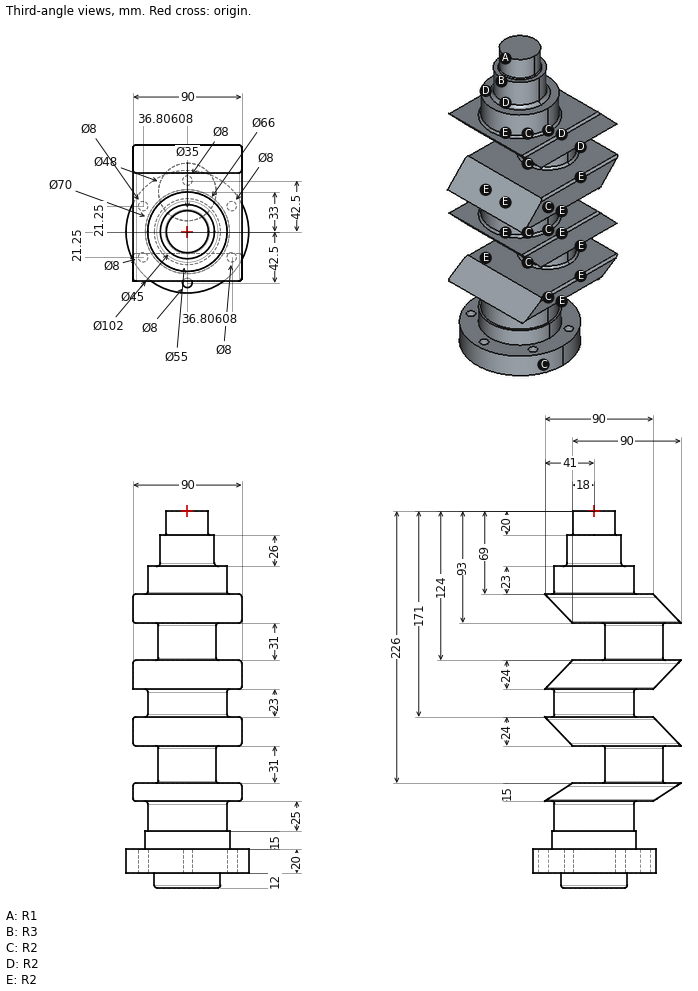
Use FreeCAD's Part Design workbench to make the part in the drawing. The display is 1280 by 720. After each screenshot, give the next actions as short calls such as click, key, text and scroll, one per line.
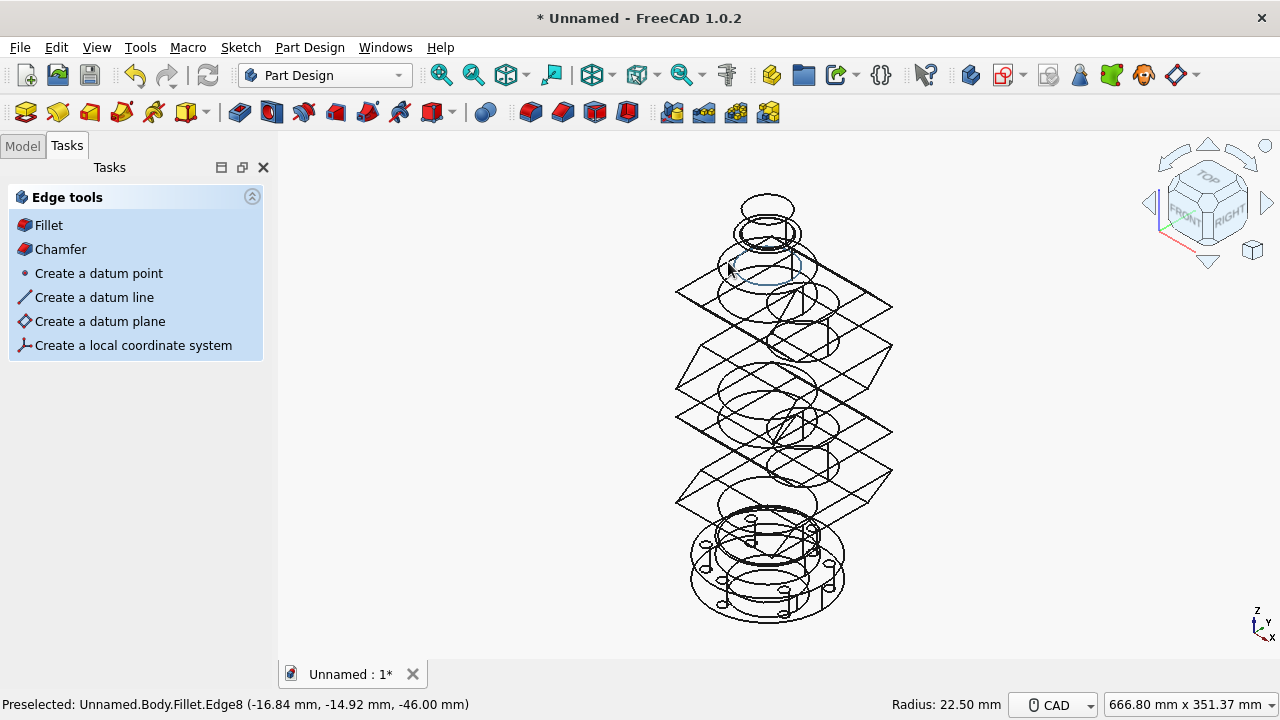
key(v)
key(1)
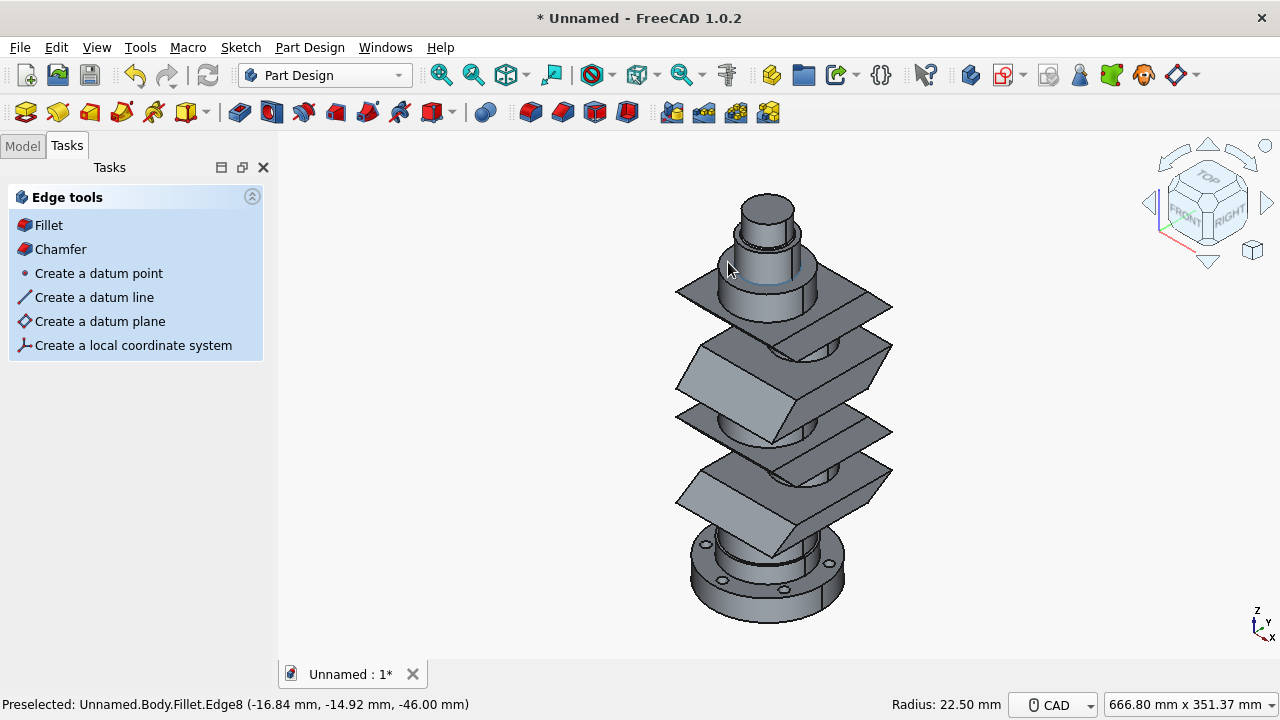
click(532, 112)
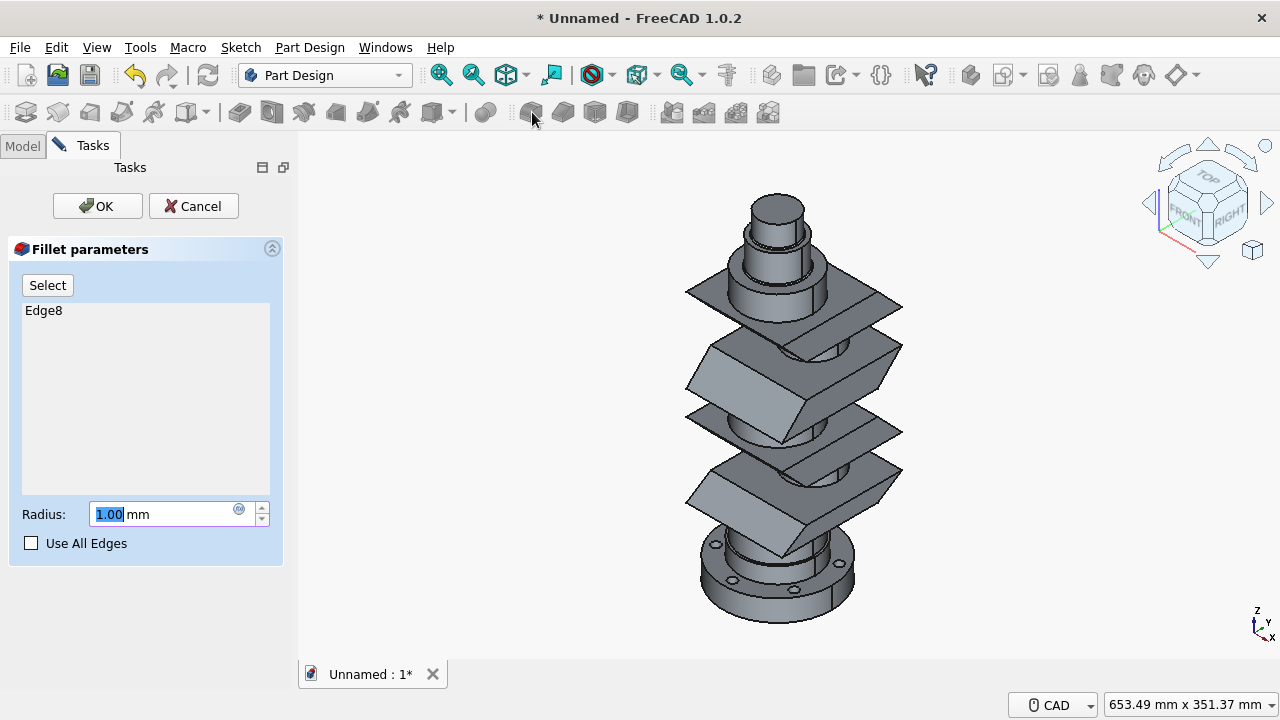
text(3)
key(Tab)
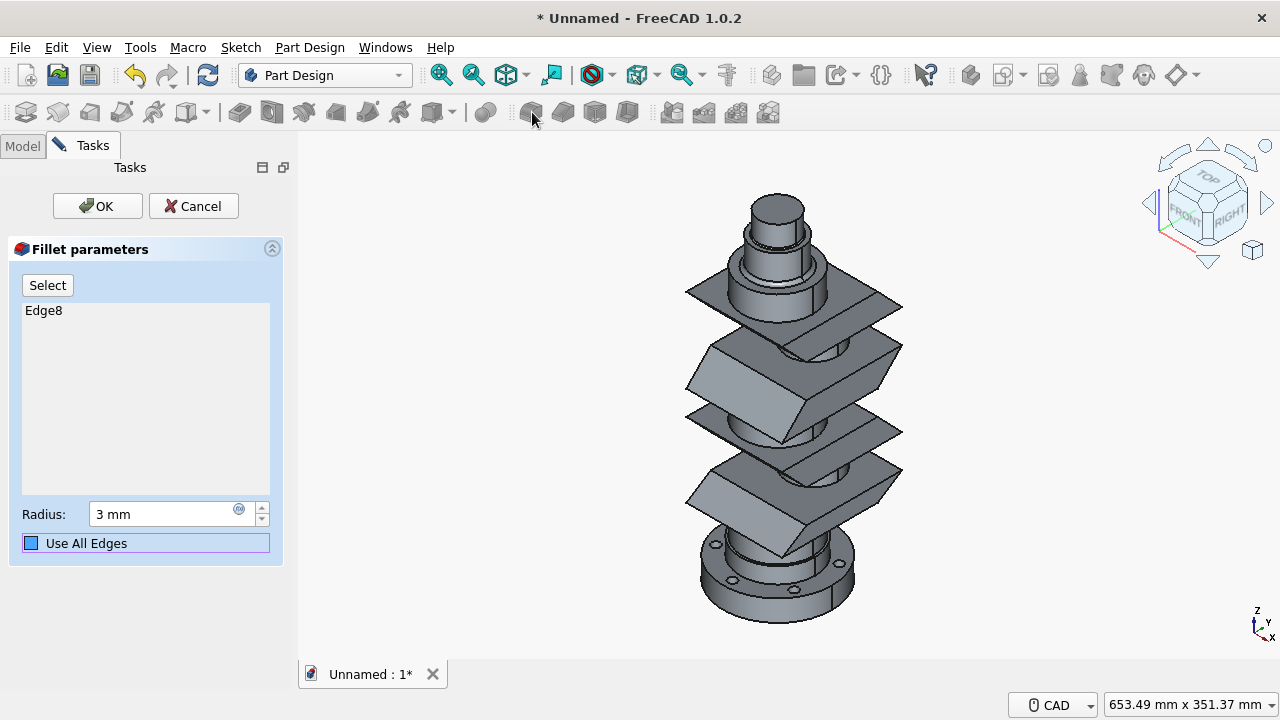
click(98, 206)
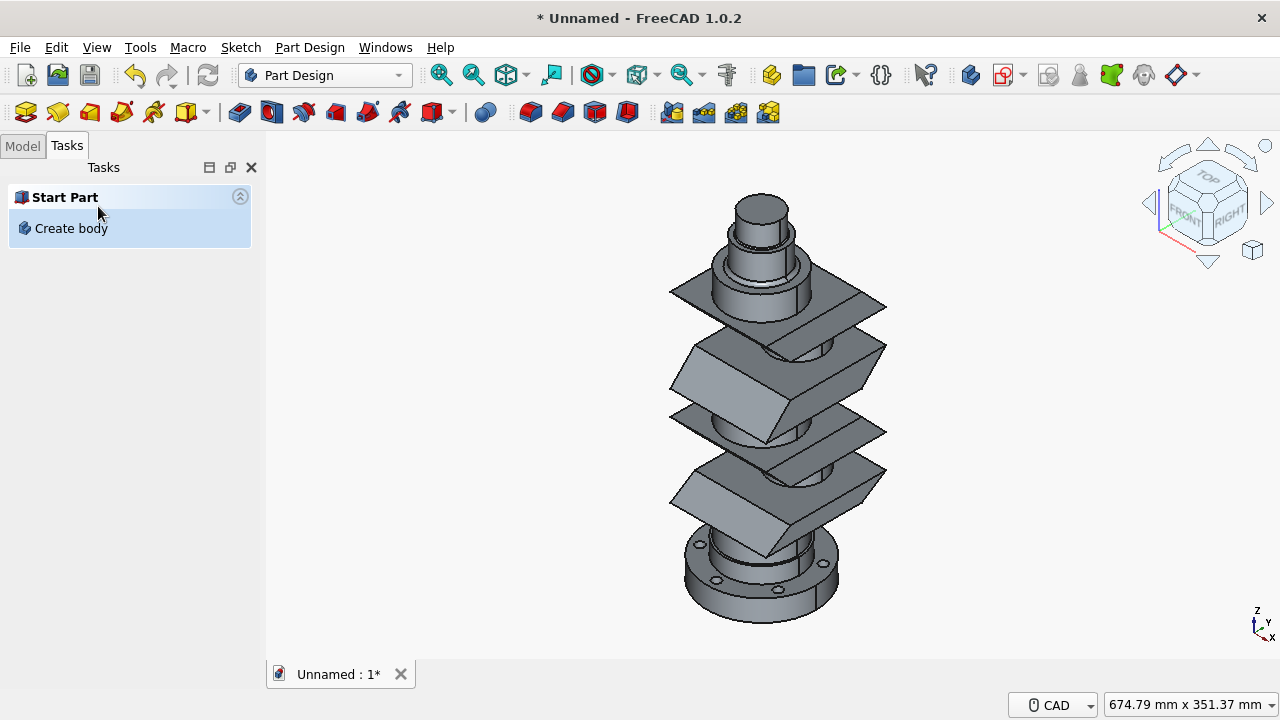
key(2)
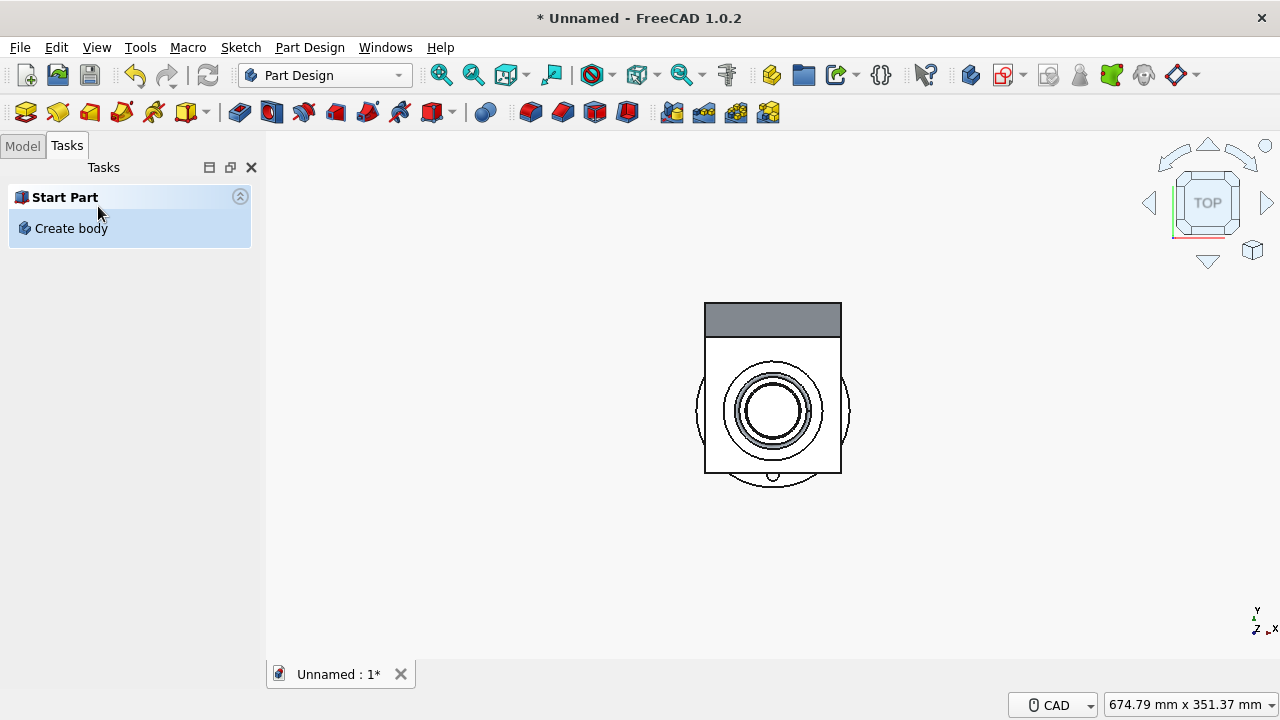
click(442, 76)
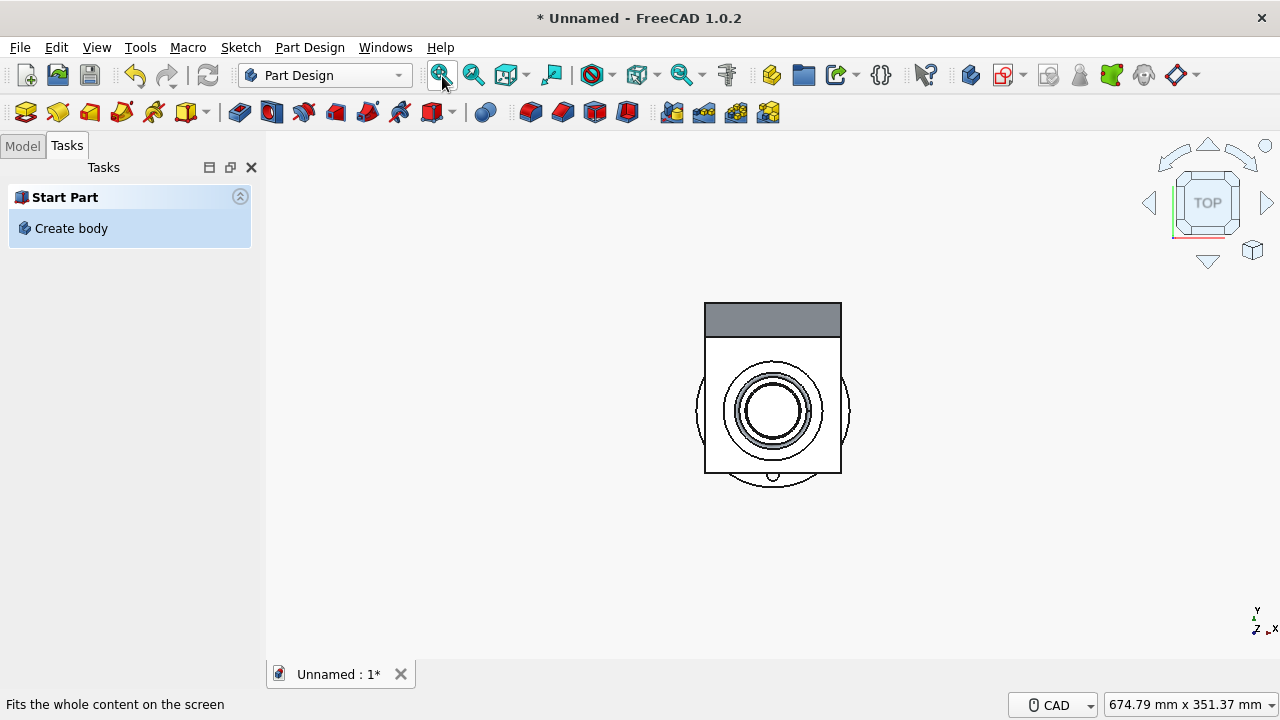
key(0)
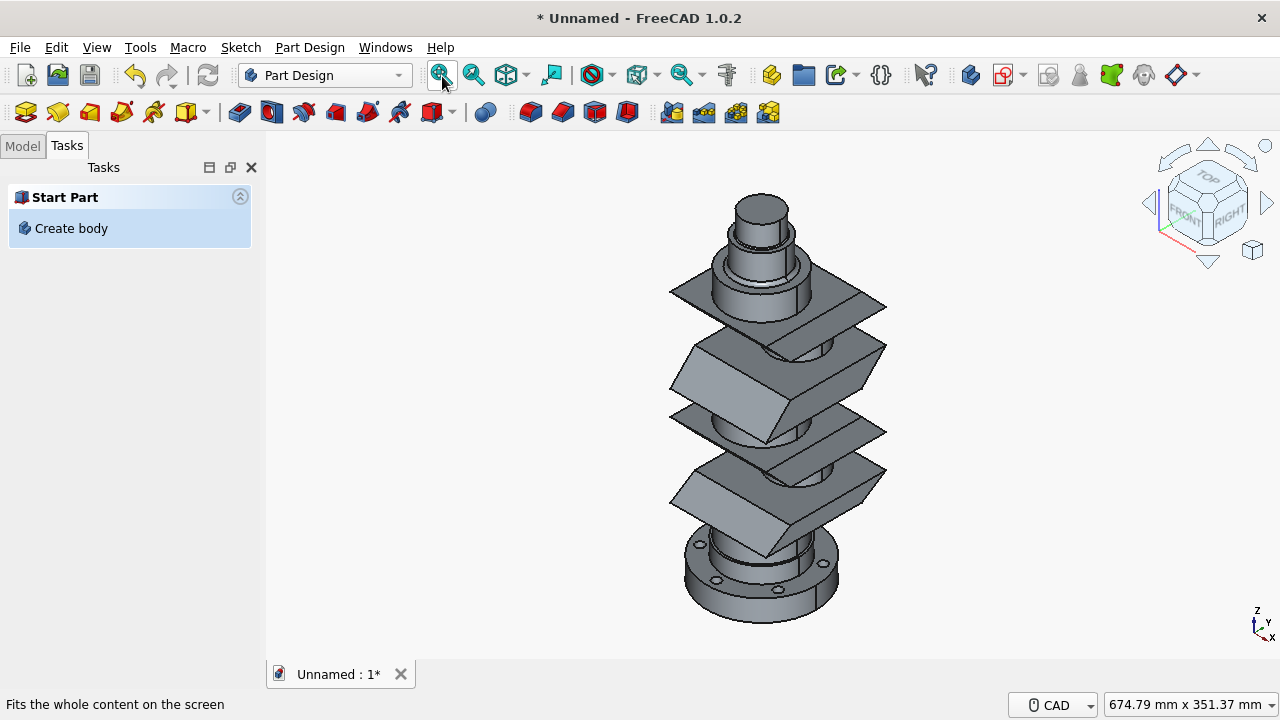
key(1)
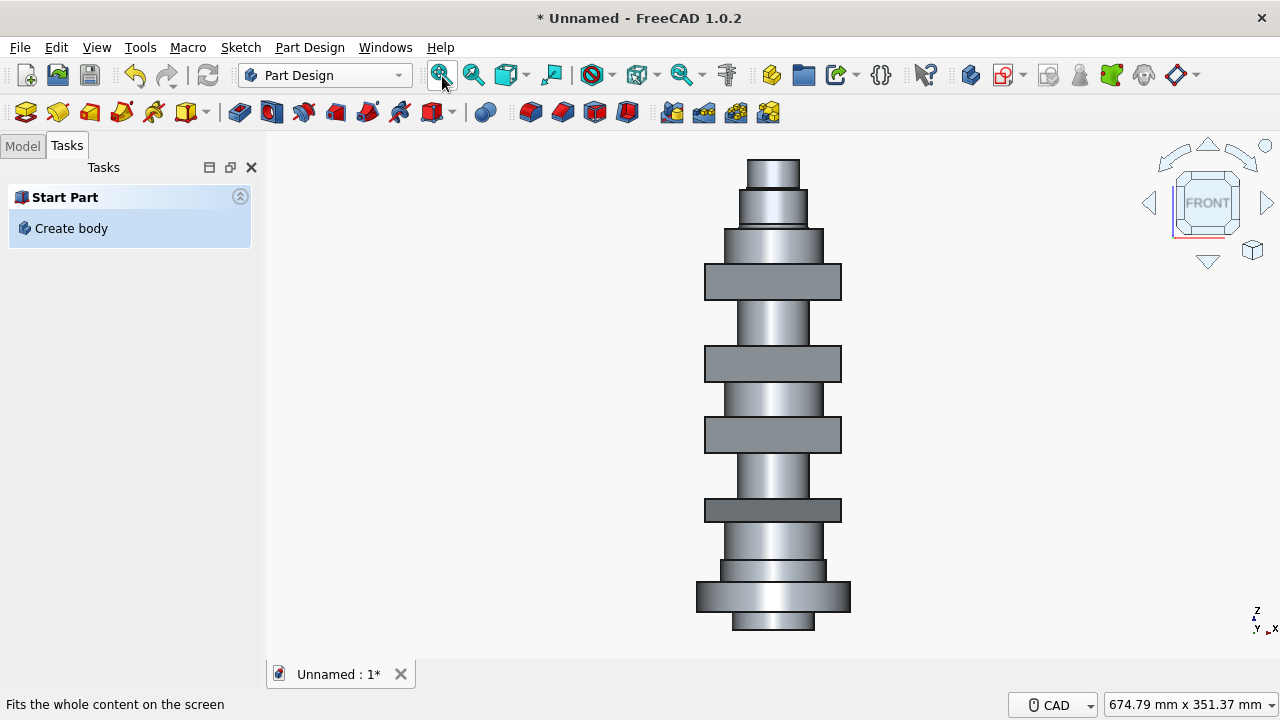
click(740, 629)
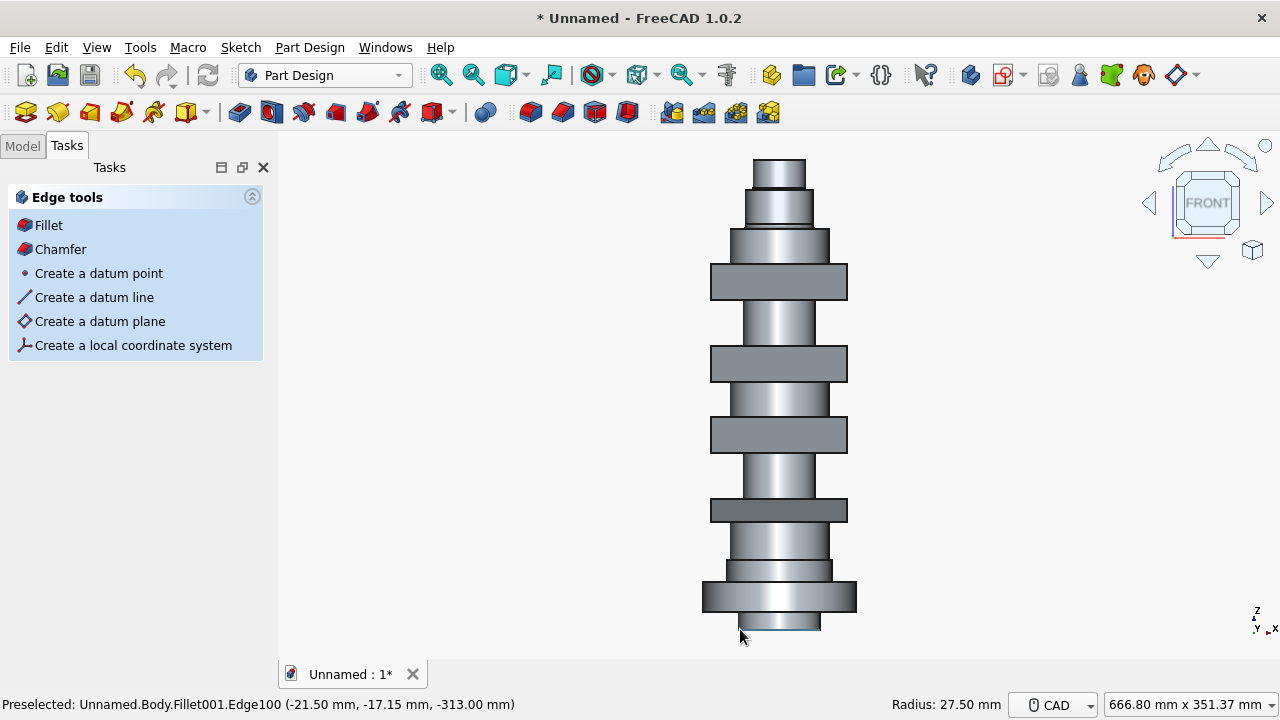
key(3)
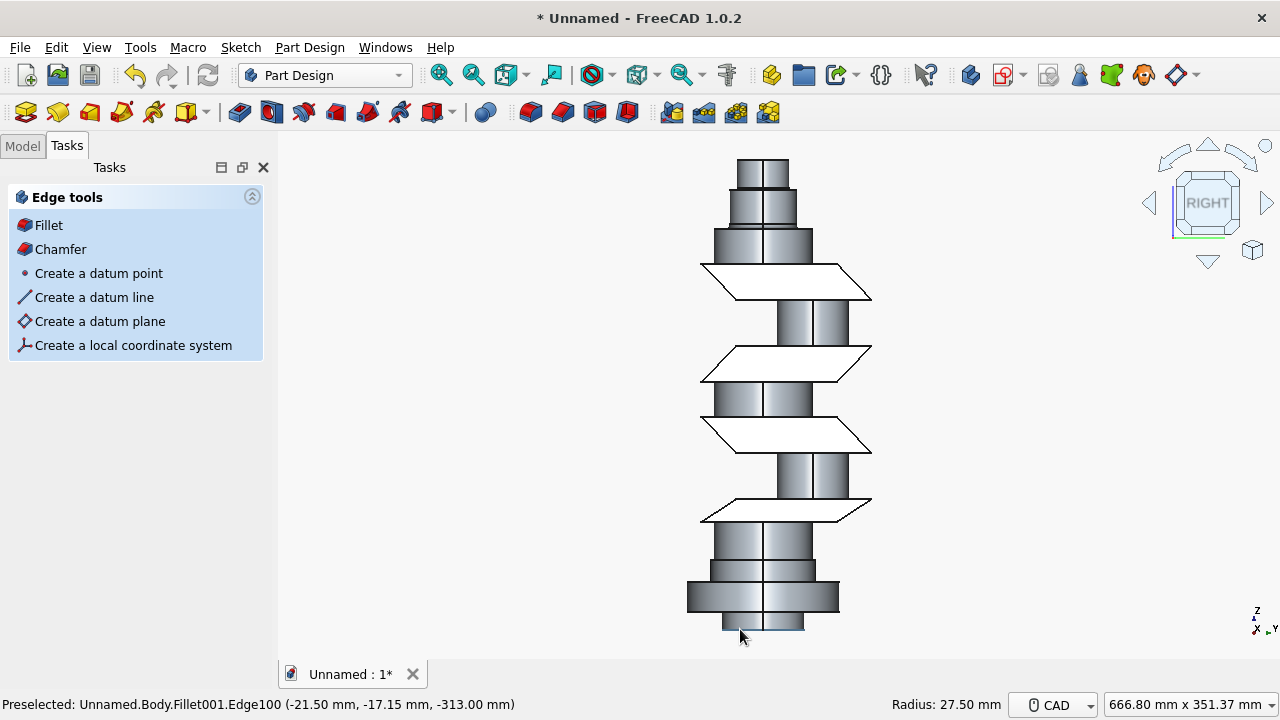
key(5)